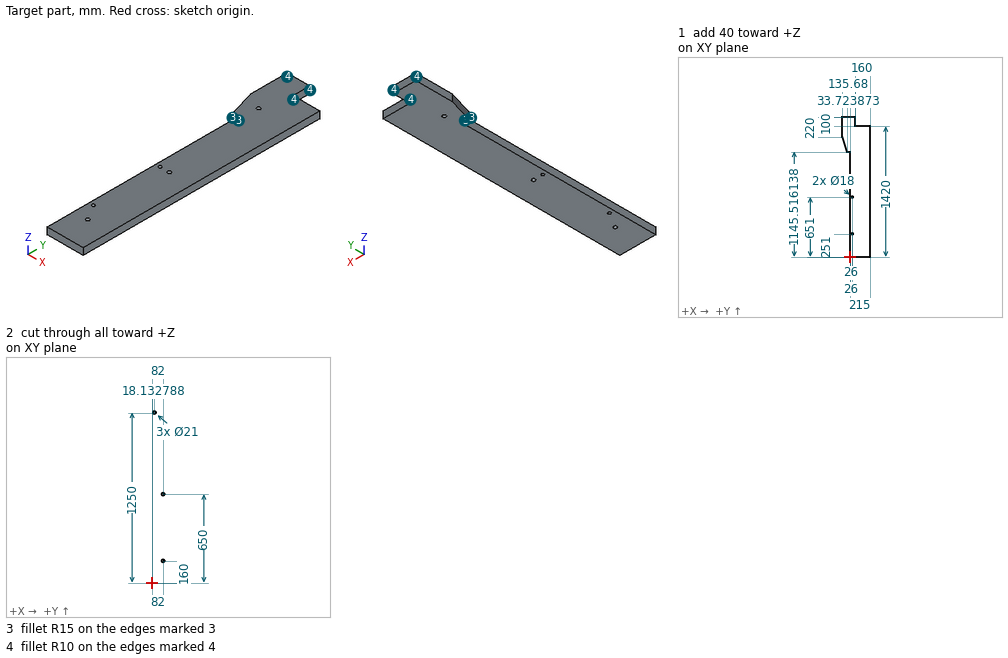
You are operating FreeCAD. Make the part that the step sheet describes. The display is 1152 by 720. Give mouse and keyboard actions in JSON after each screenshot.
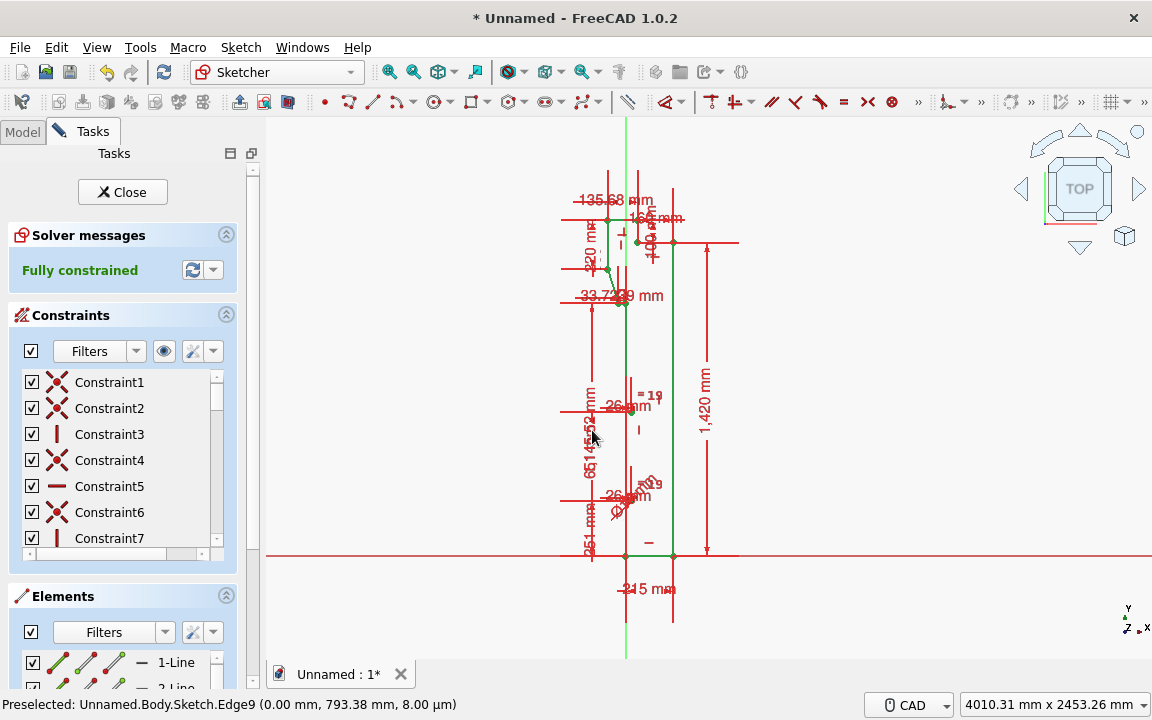
{"action": "left_click", "coordinate": [123, 192]}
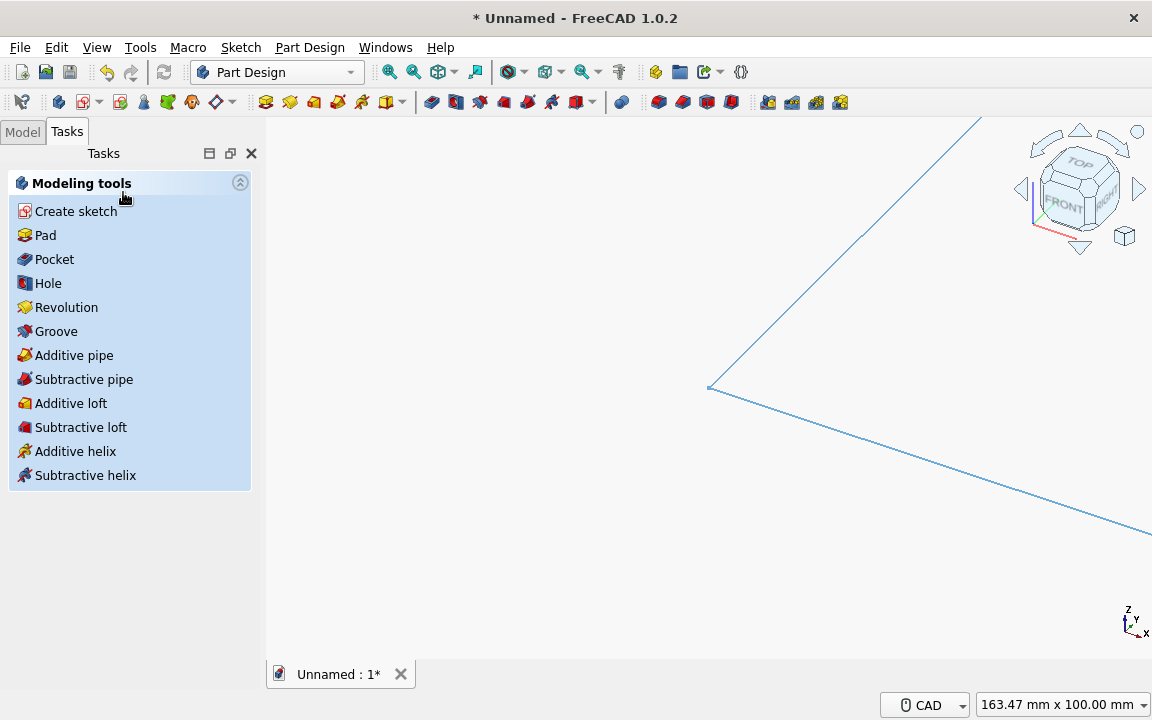
{"action": "left_click", "coordinate": [266, 102]}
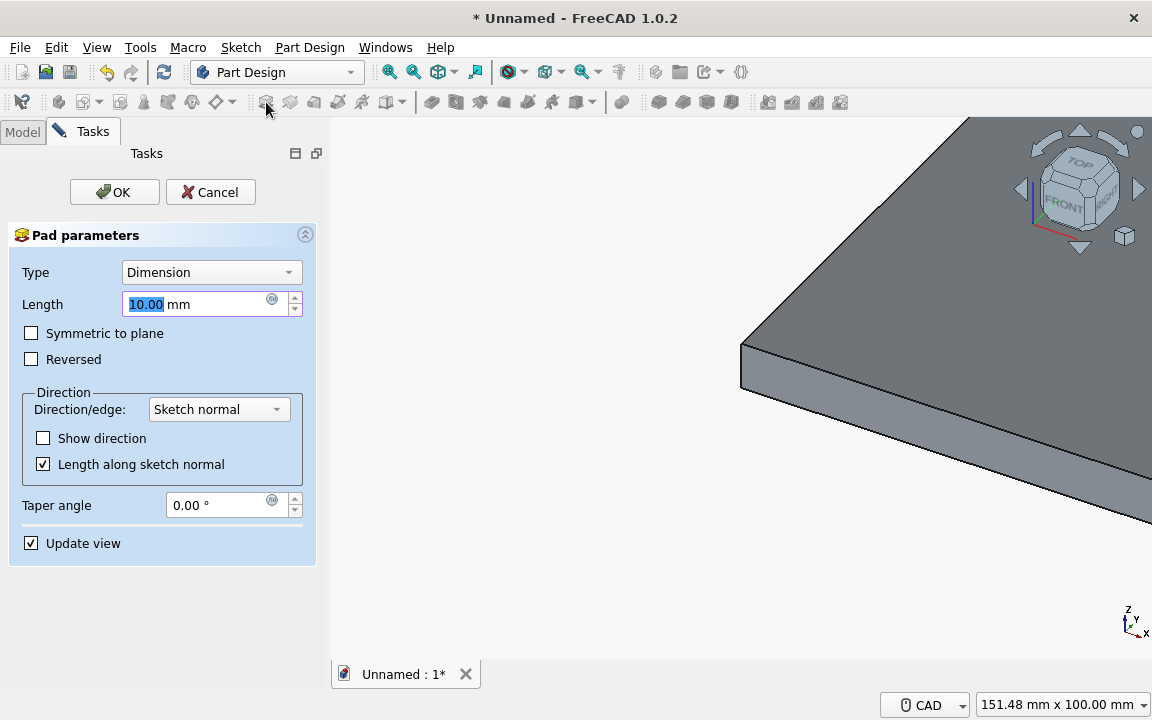
{"action": "type", "text": "40"}
{"action": "key", "text": "Tab"}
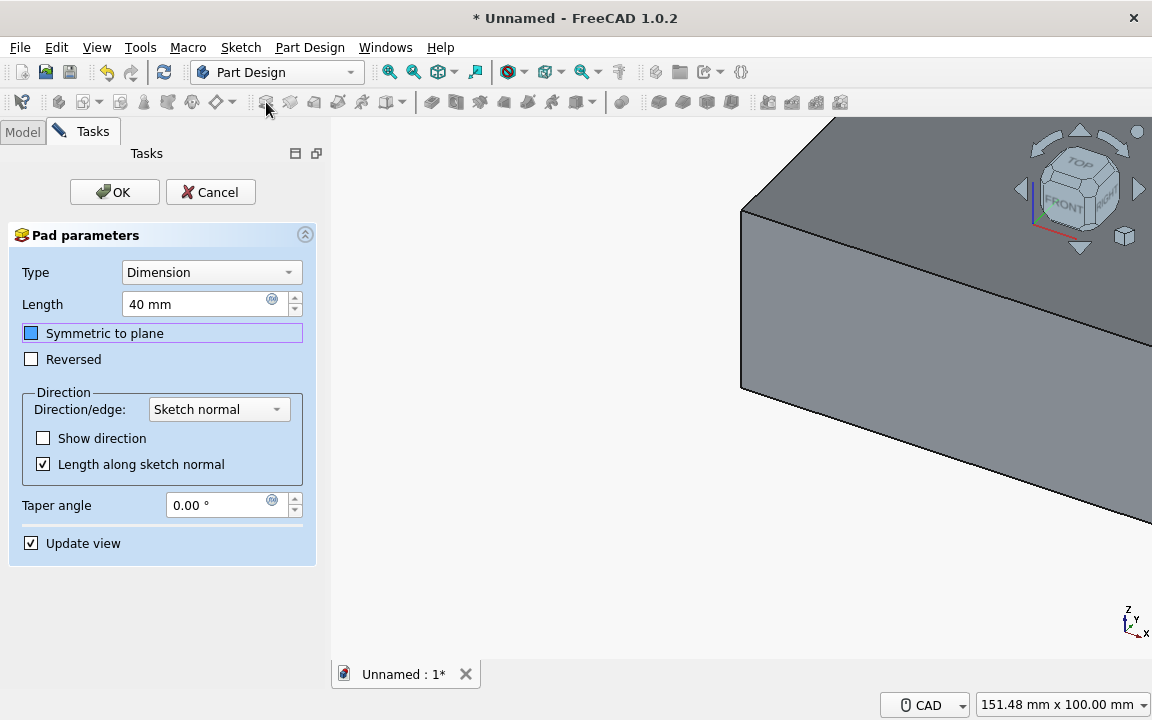
{"action": "left_click", "coordinate": [115, 192]}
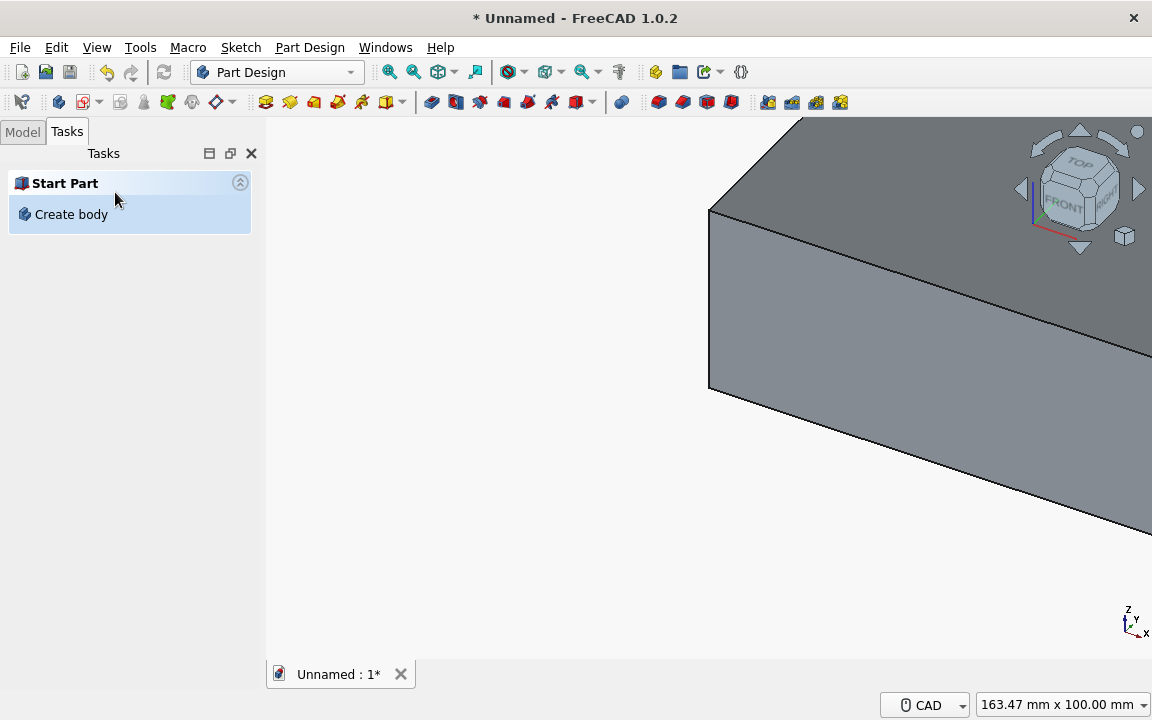
{"action": "left_click", "coordinate": [390, 72]}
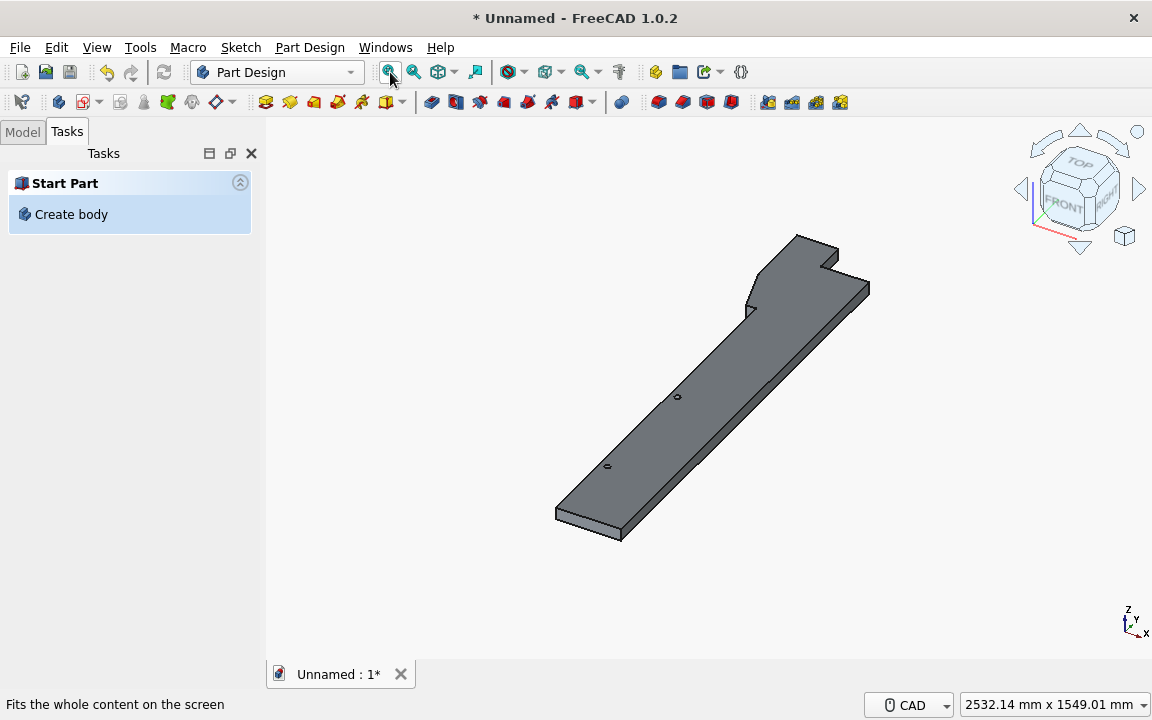
{"action": "left_click", "coordinate": [84, 102]}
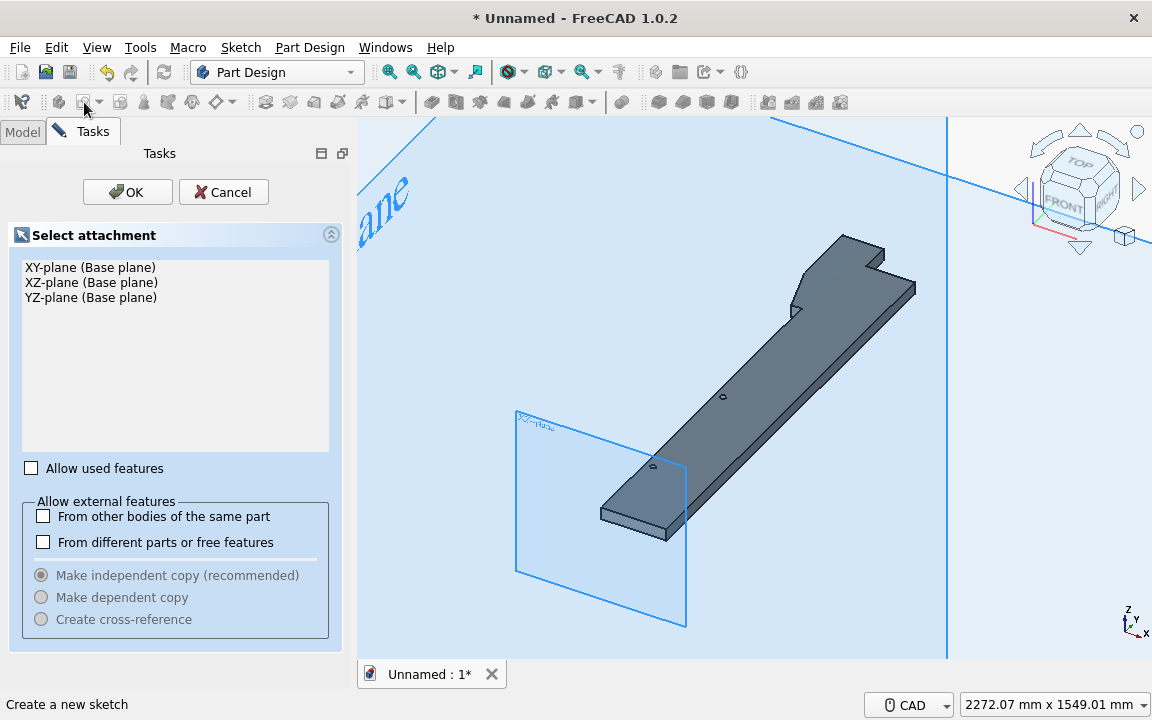
{"action": "left_click", "coordinate": [82, 268]}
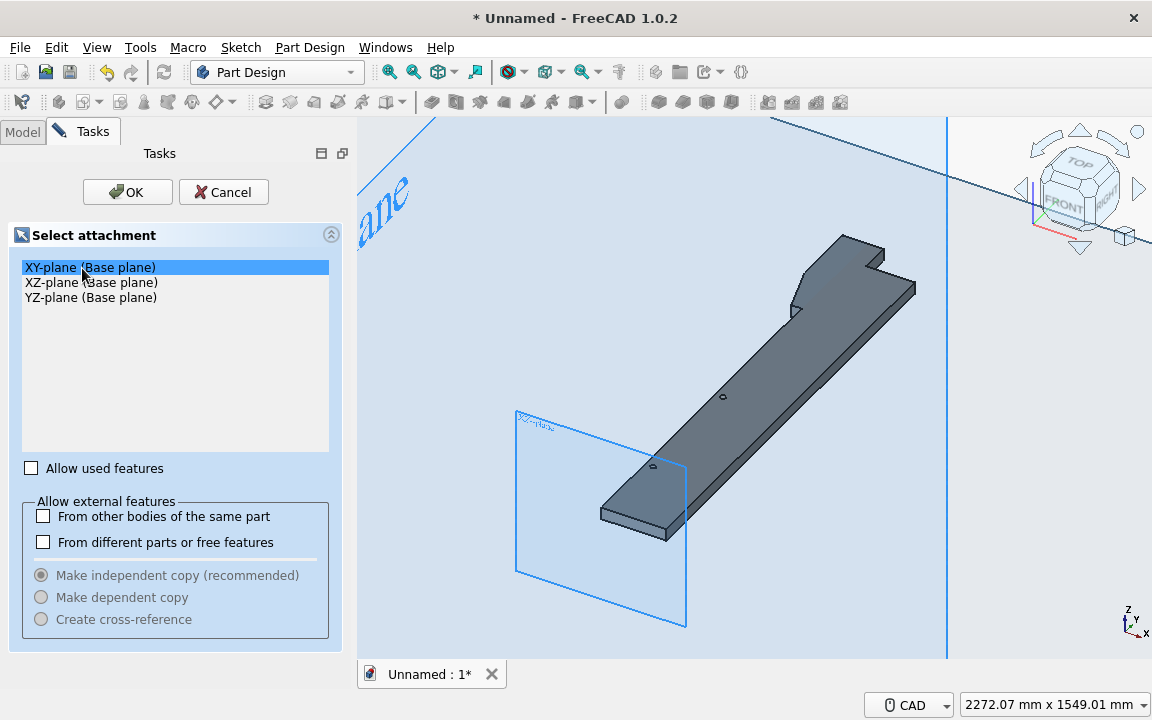
{"action": "left_click", "coordinate": [128, 192]}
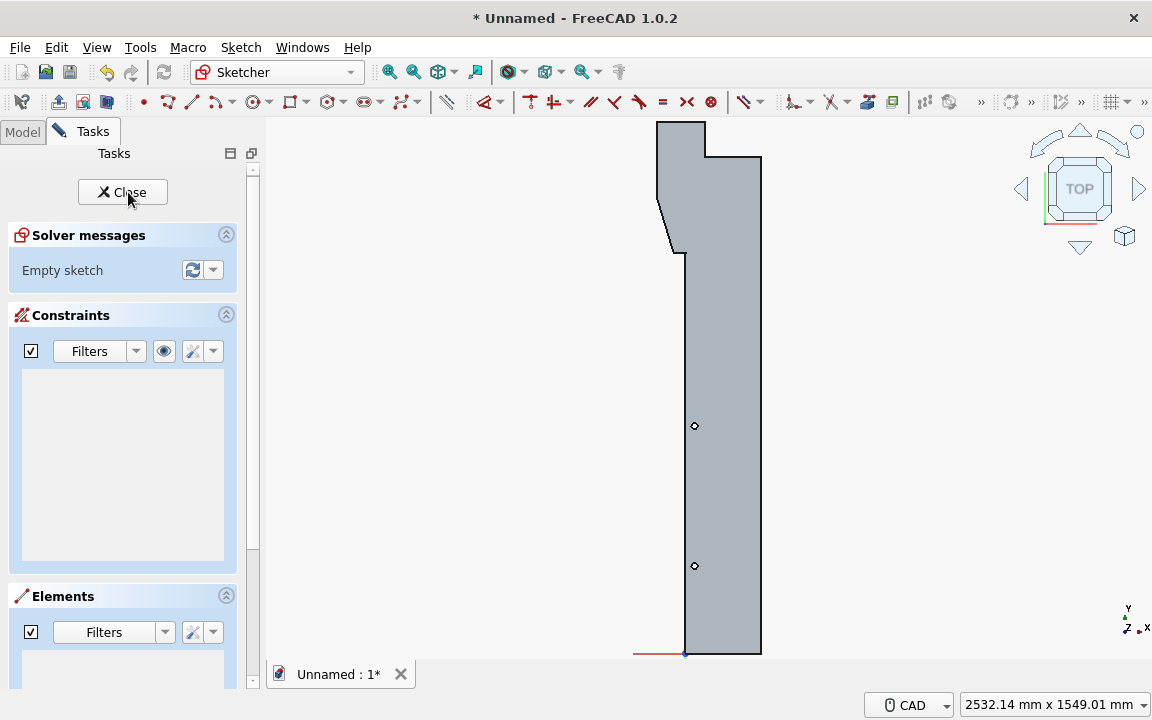
{"action": "key", "text": "q s"}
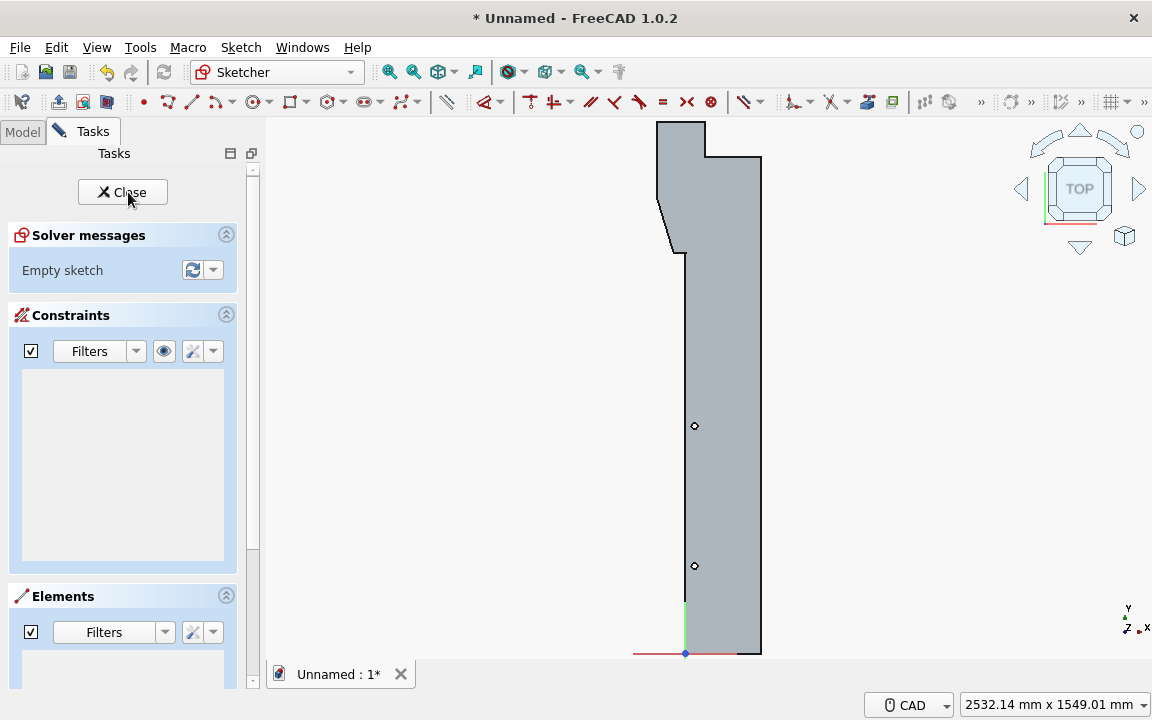
{"action": "scroll", "coordinate": [364, 183], "scroll_direction": "down", "scroll_amount": 1}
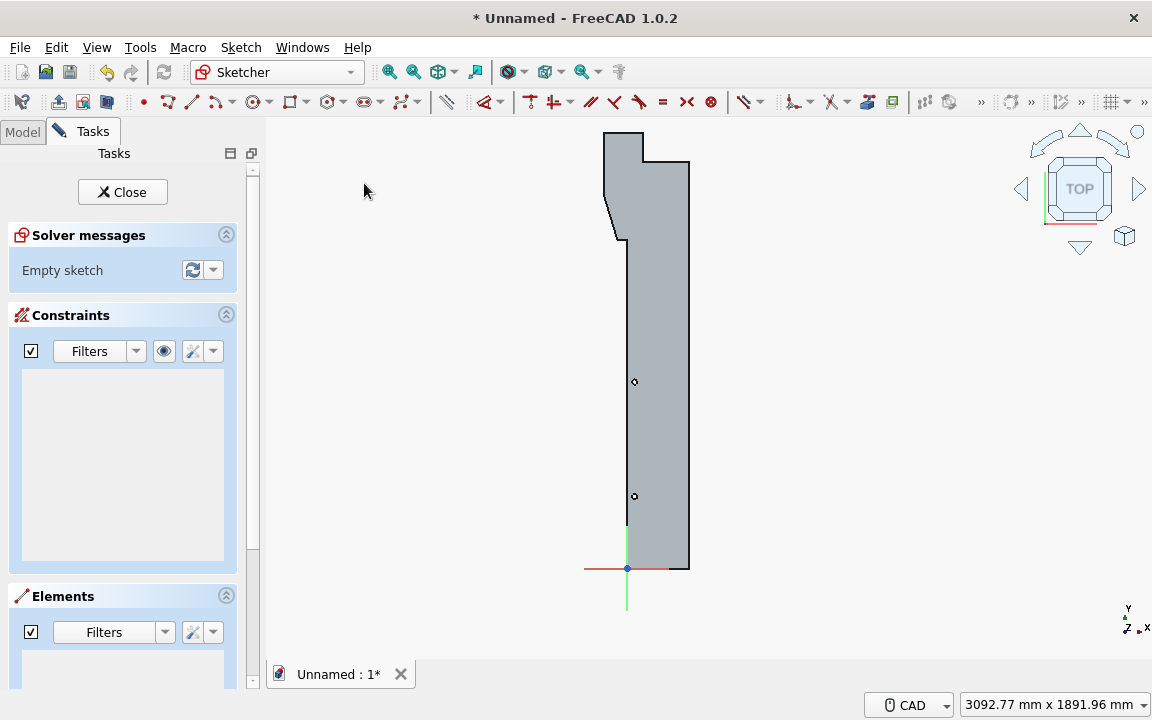
{"action": "left_click", "coordinate": [254, 102]}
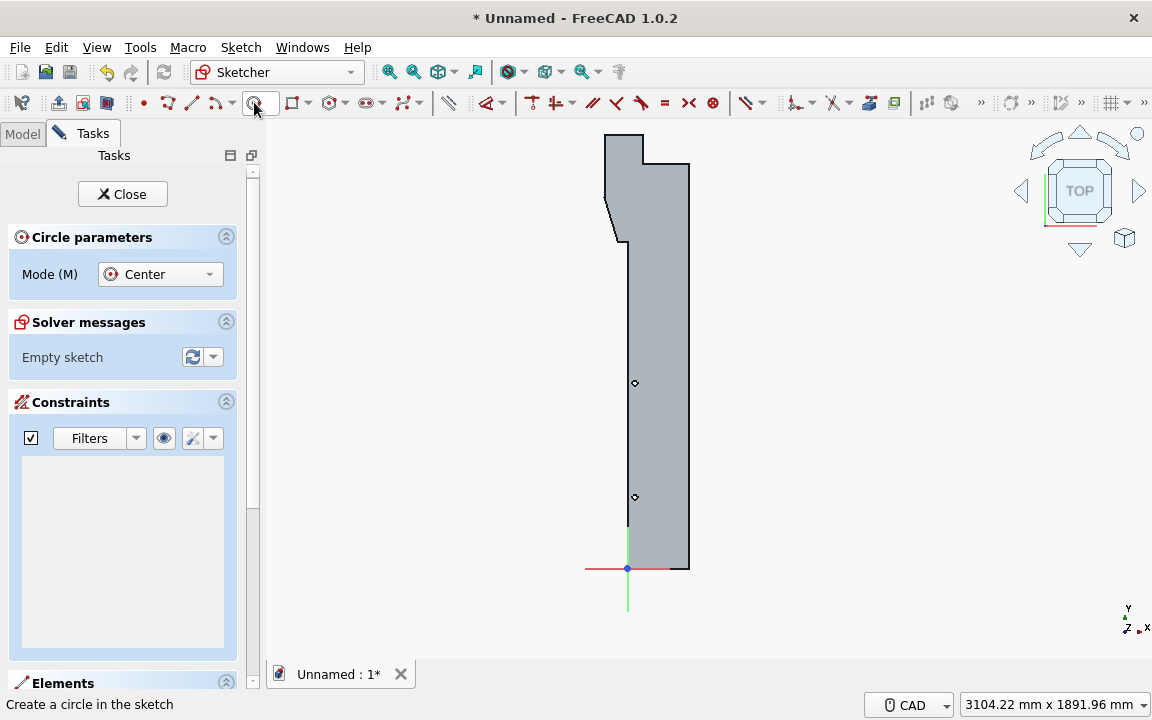
{"action": "scroll", "coordinate": [633, 212], "scroll_direction": "up", "scroll_amount": 11}